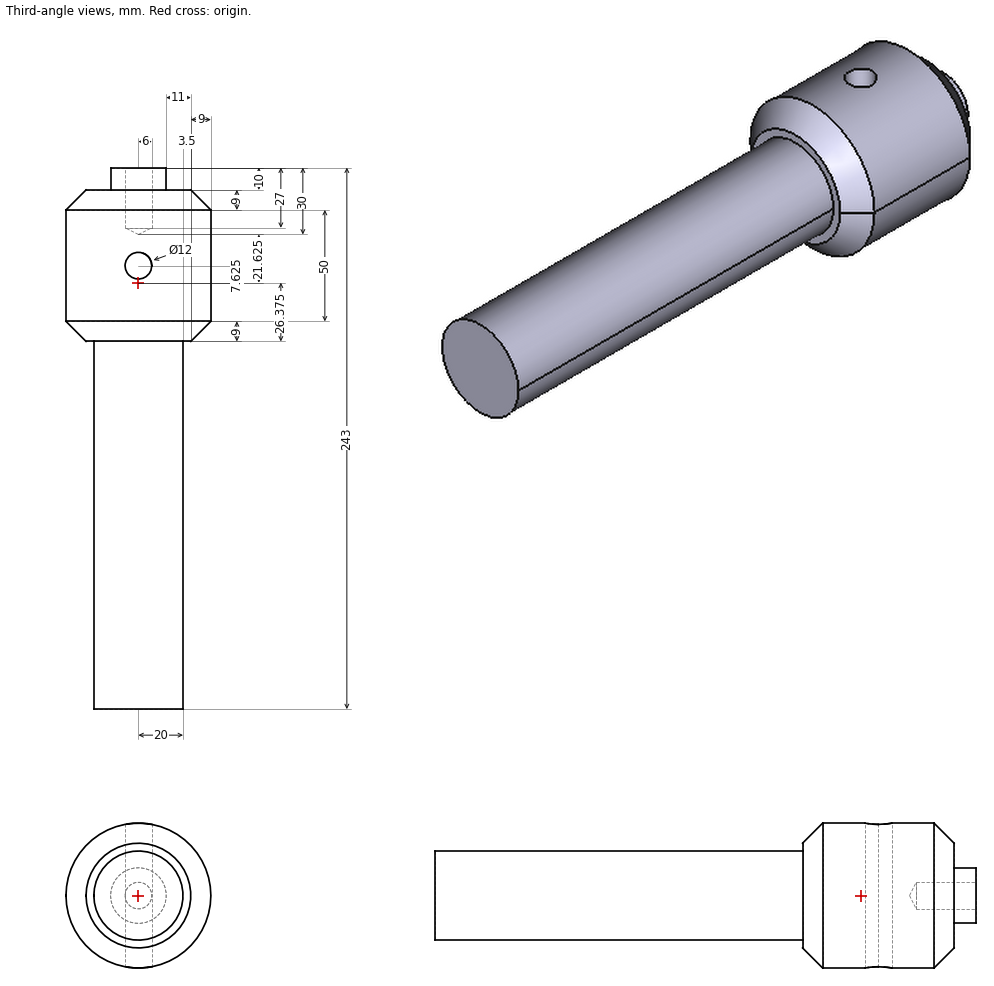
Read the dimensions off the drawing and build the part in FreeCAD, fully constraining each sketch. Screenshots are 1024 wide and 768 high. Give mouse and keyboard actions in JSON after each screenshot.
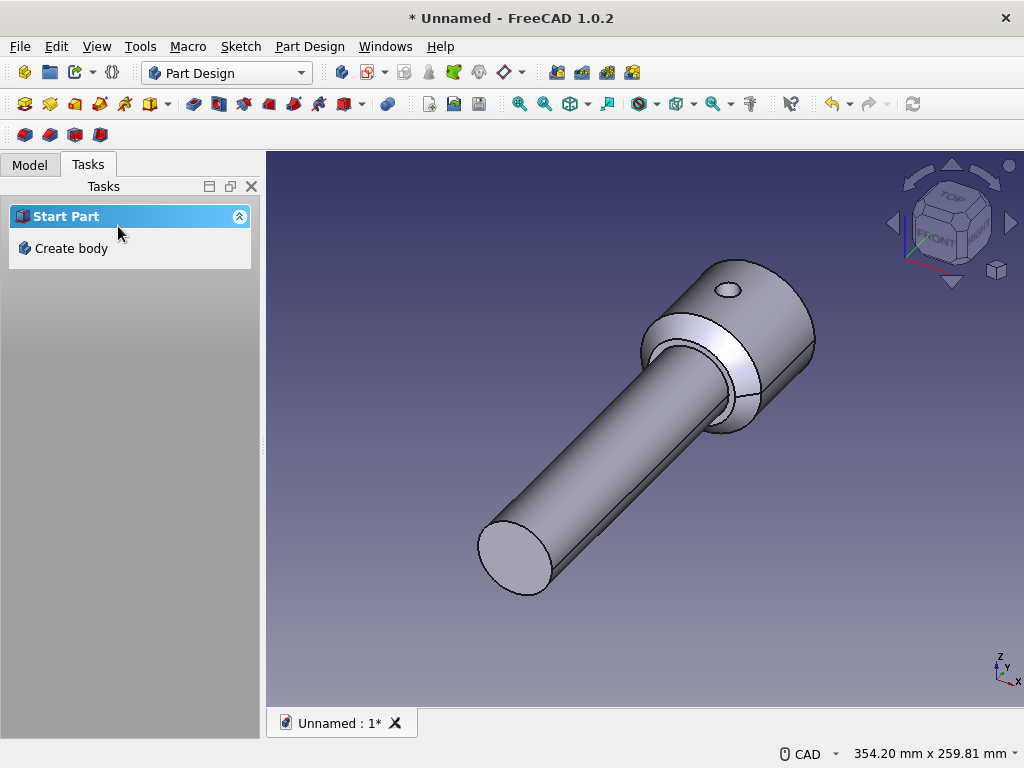
{"action": "key", "text": "0"}